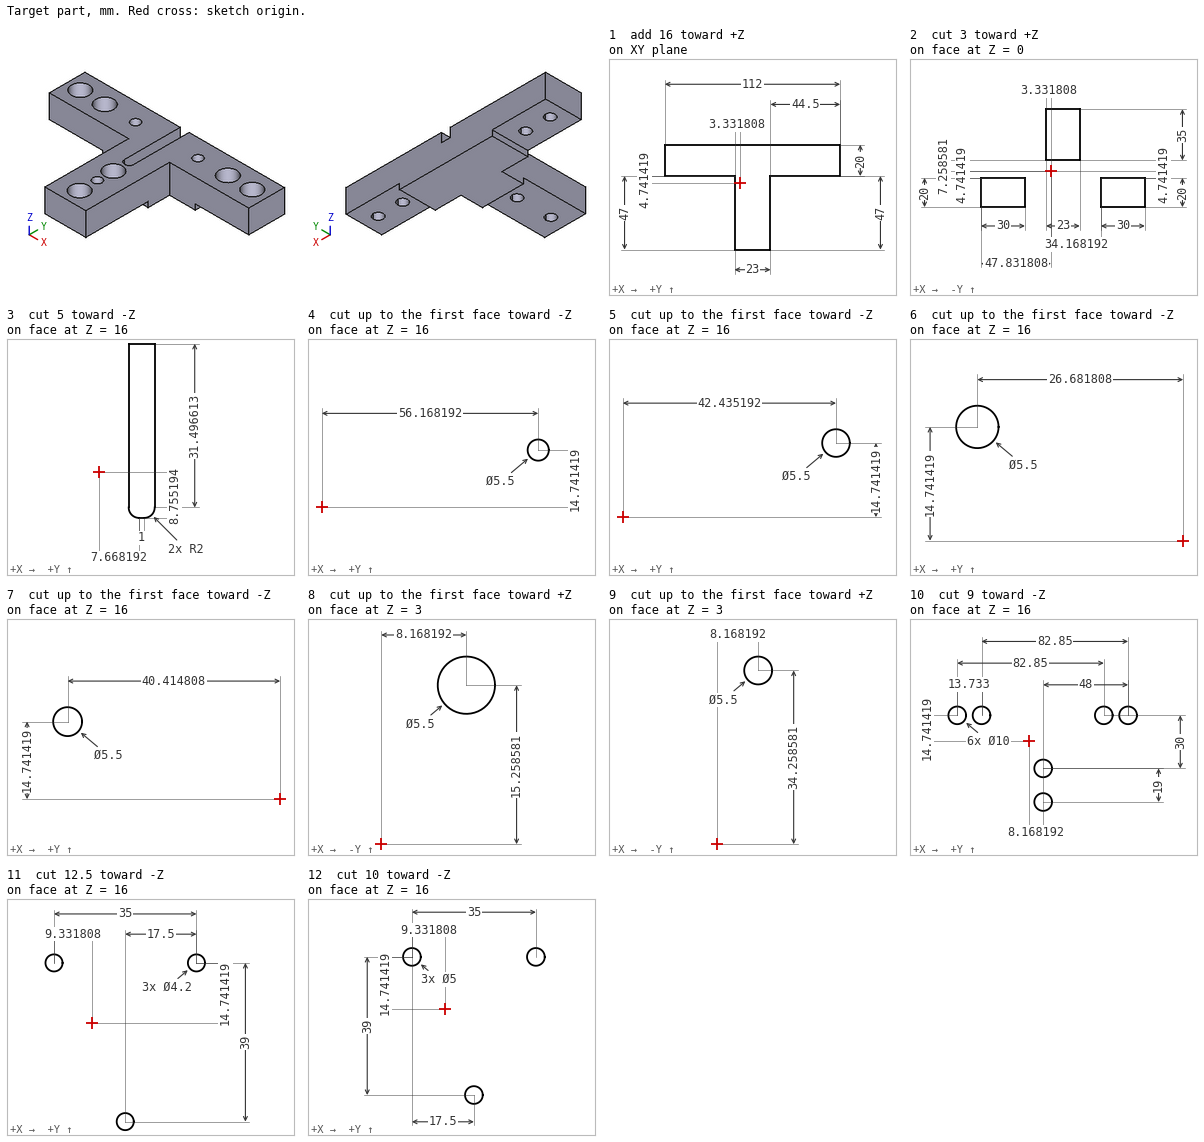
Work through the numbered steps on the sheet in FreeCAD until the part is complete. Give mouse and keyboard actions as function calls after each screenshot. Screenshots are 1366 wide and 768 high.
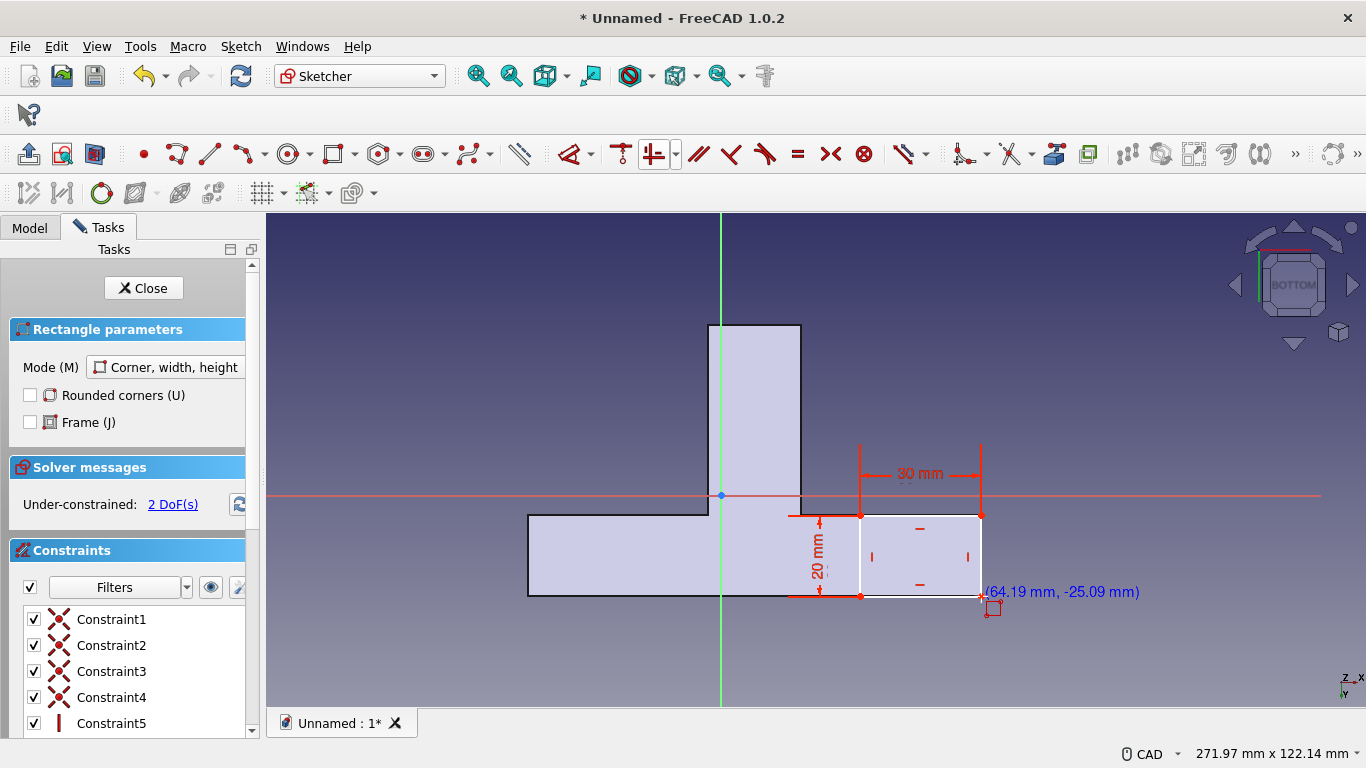
click(708, 325)
move(801, 466)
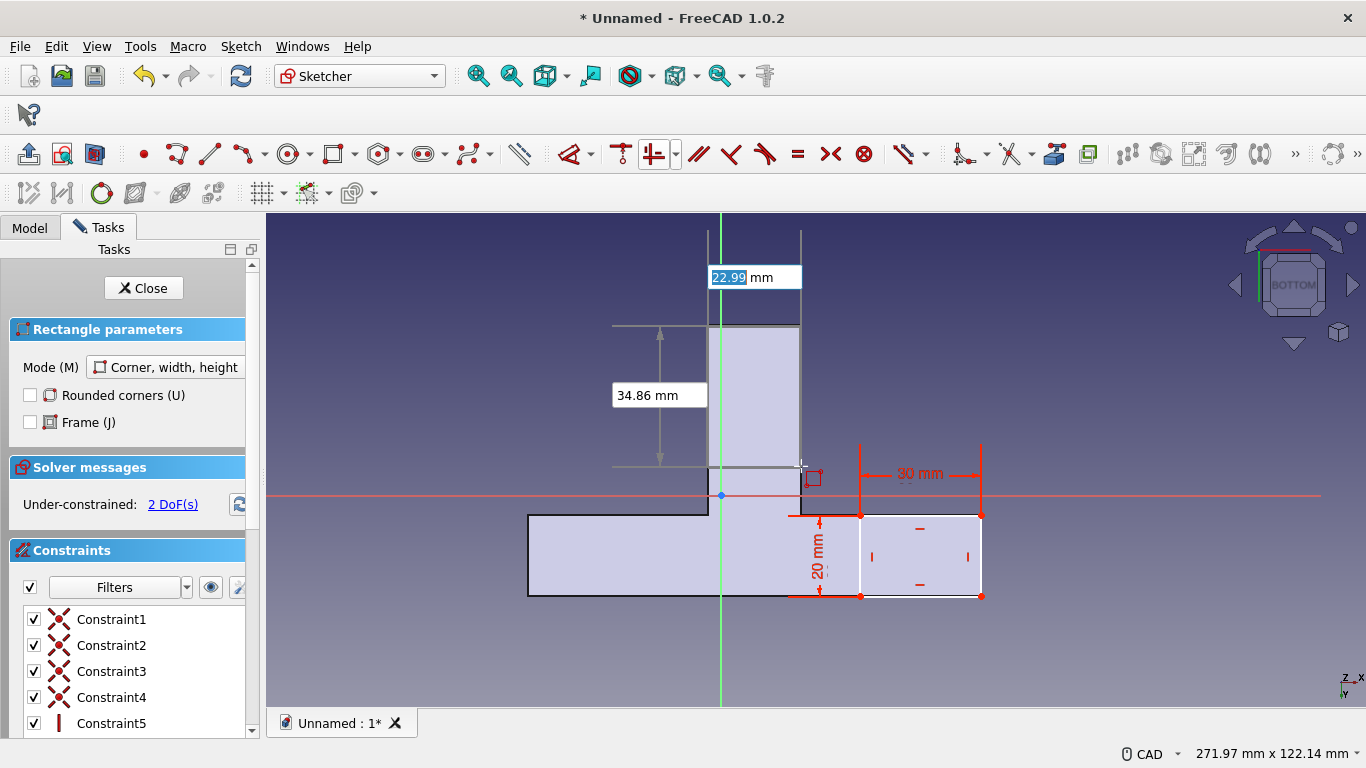
text(23)
key(Tab)
text(35)
key(Return)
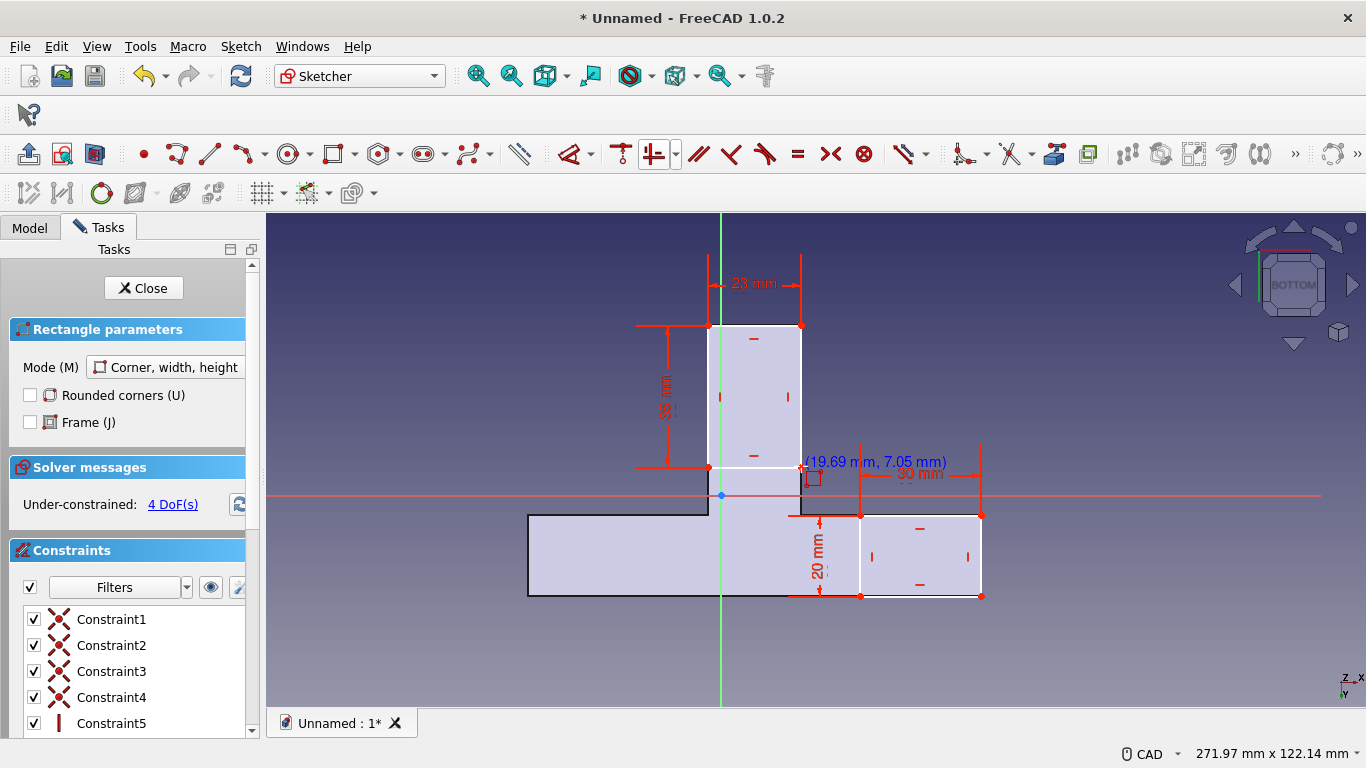
click(528, 515)
move(649, 596)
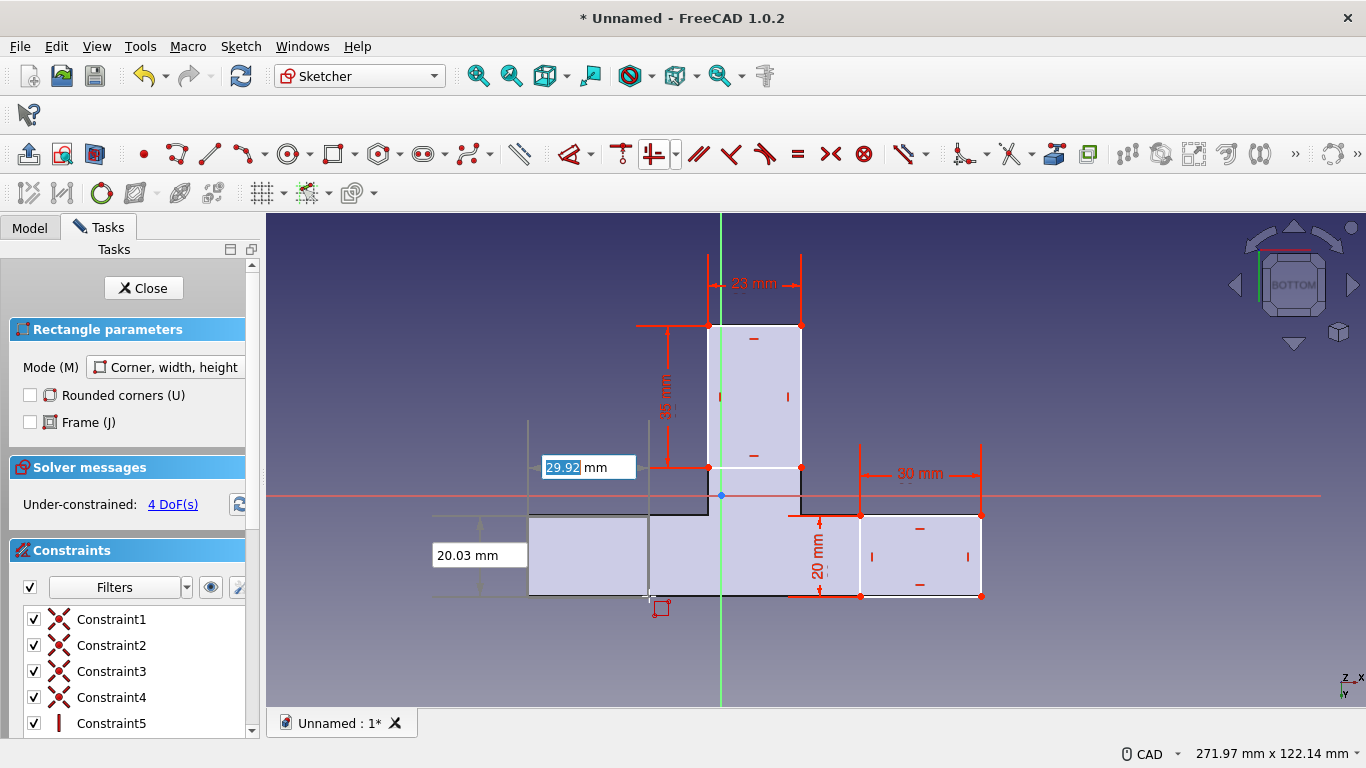
text(30)
key(Tab)
text(20)
key(Return)
key(Escape)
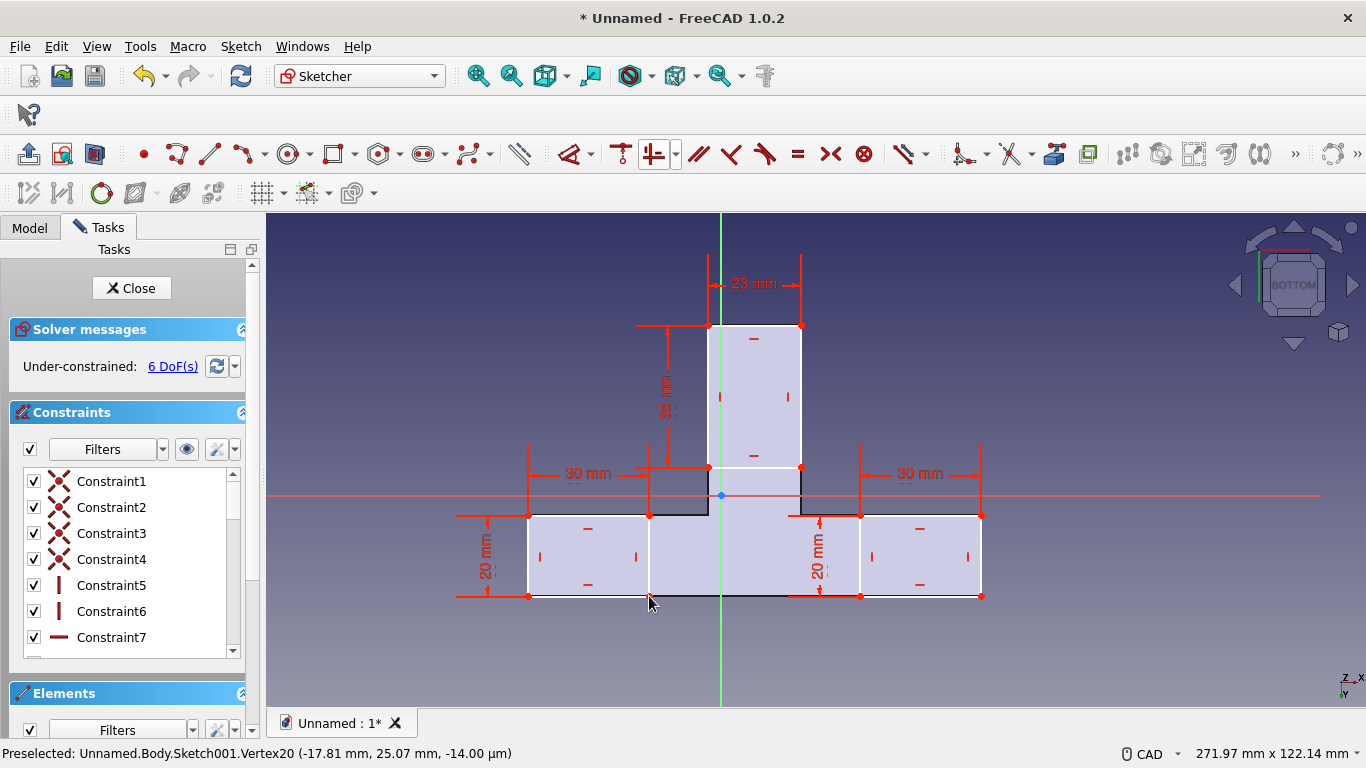
click(568, 154)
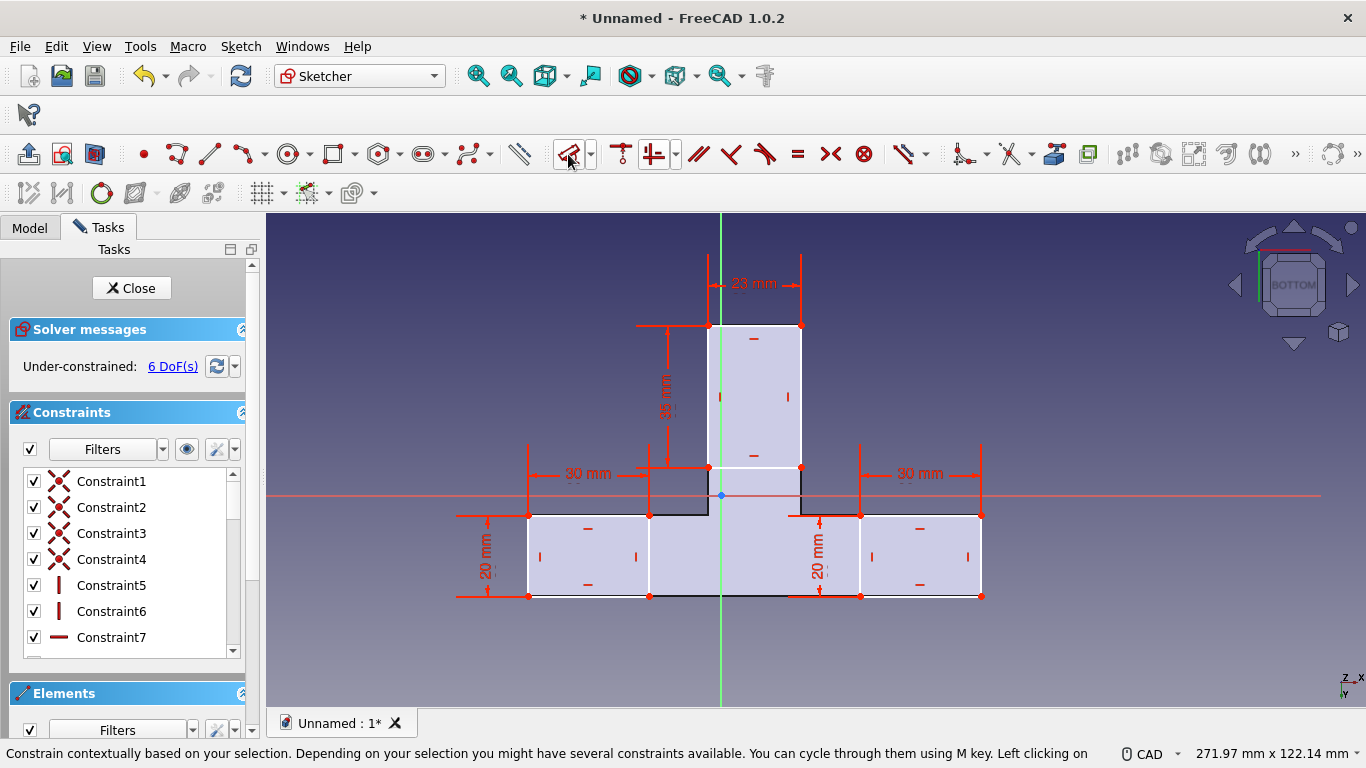
scroll(860, 516, up, 4)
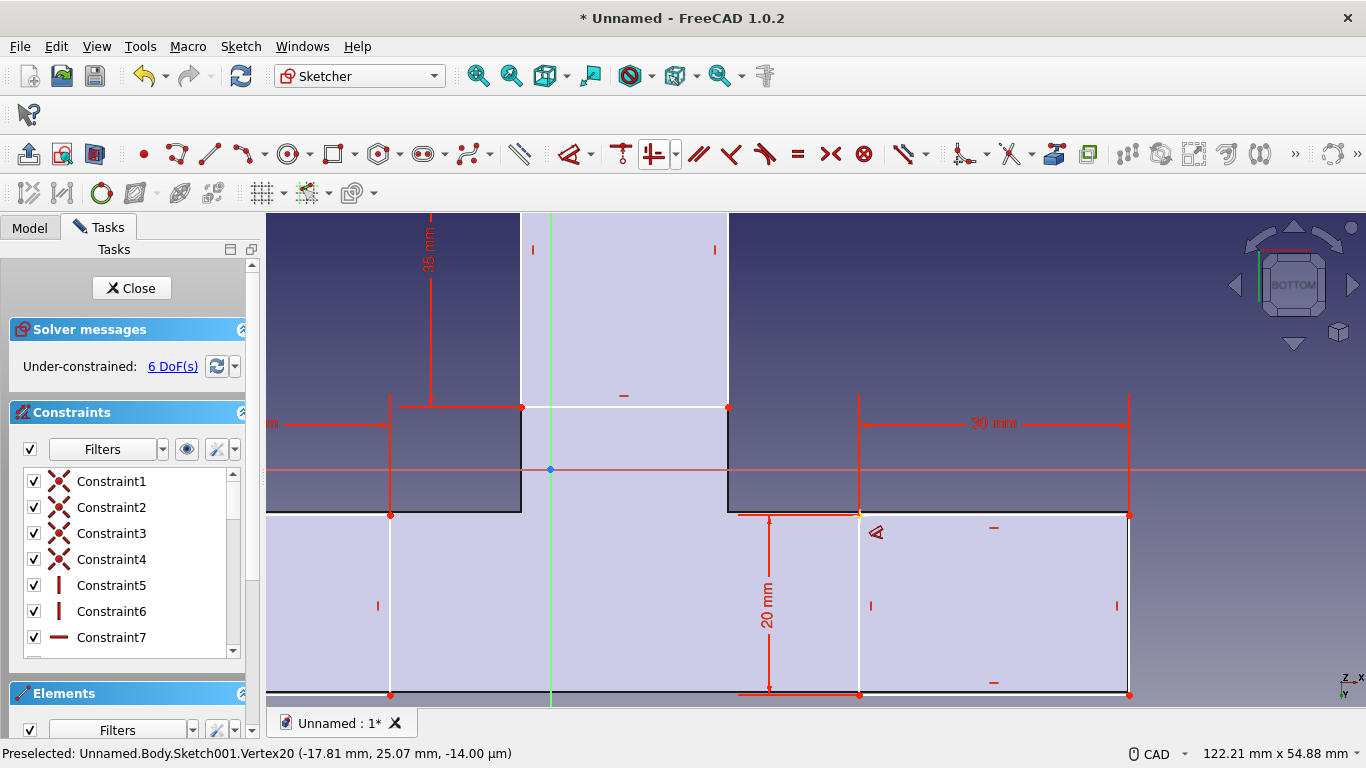
click(859, 515)
click(893, 492)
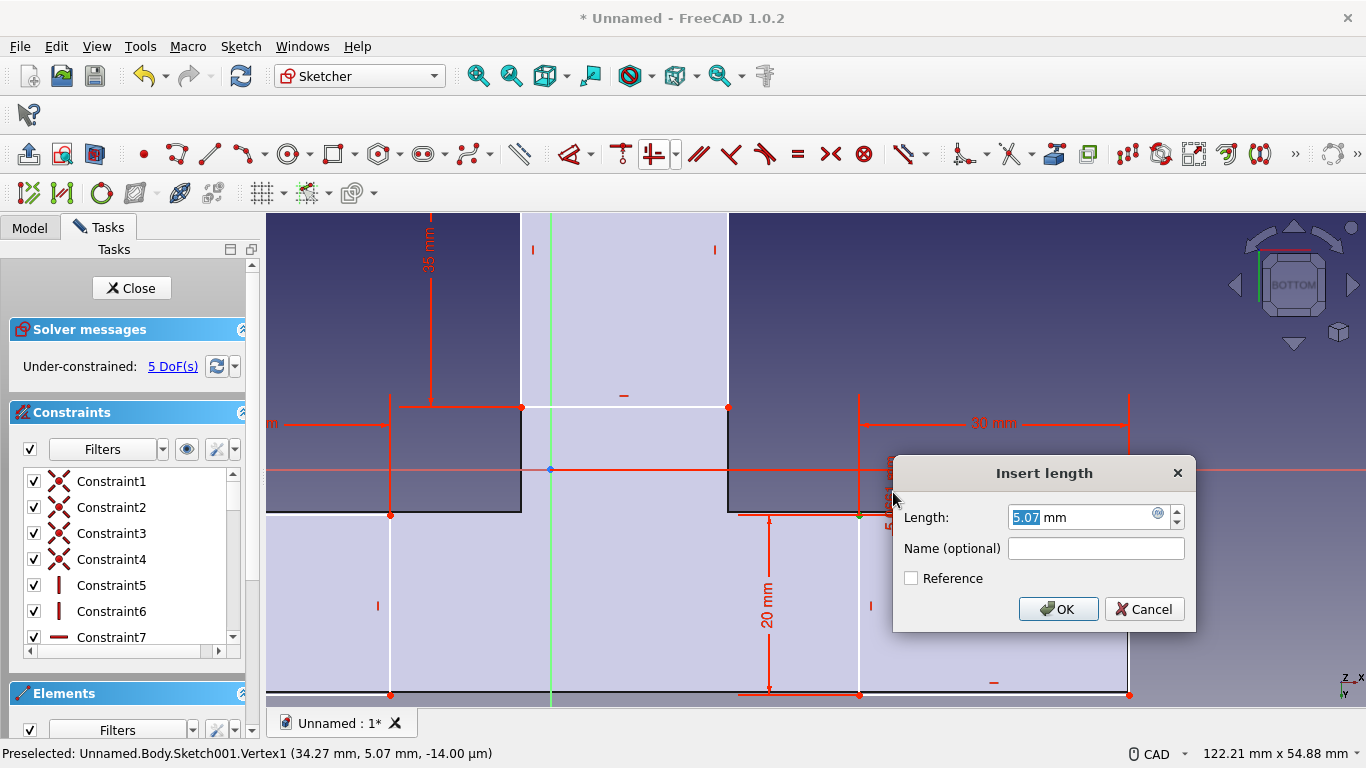
text(4.741419)
key(Return)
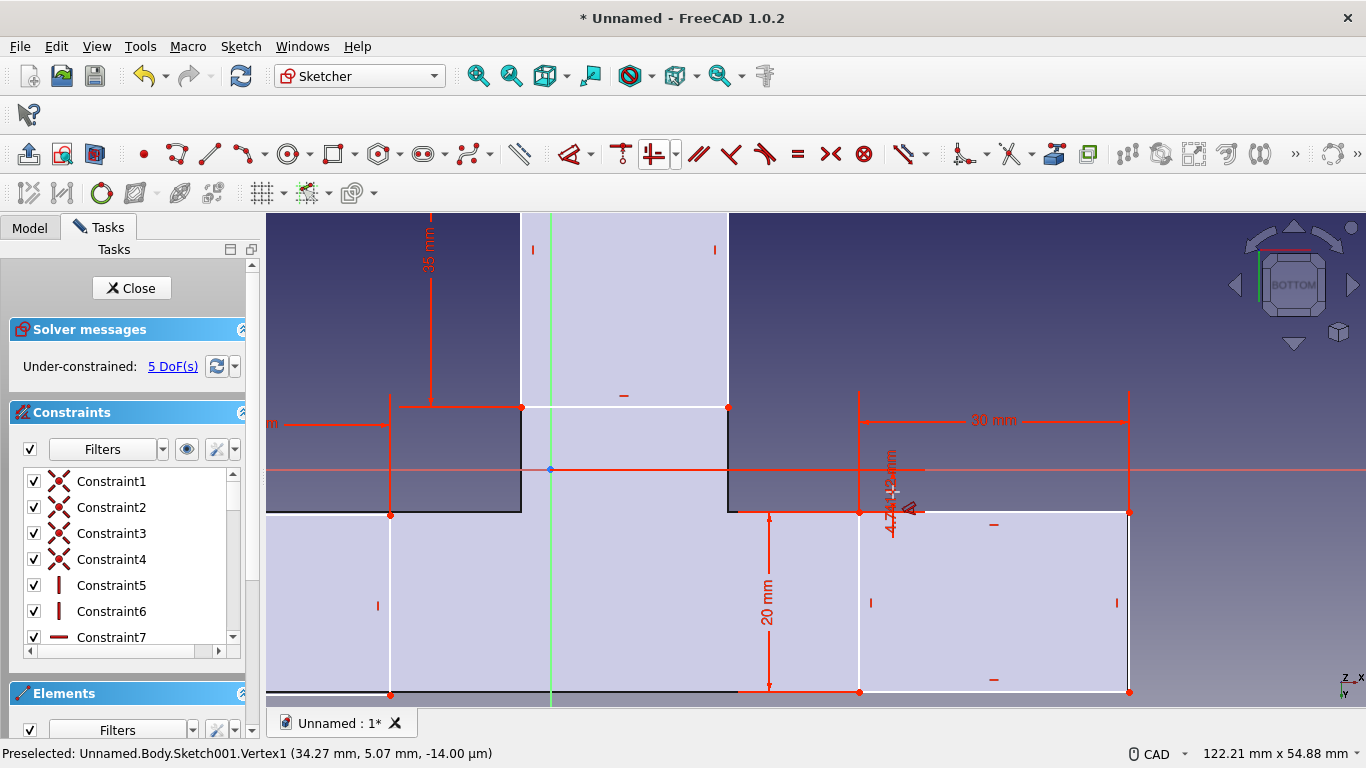
scroll(897, 544, down, 3)